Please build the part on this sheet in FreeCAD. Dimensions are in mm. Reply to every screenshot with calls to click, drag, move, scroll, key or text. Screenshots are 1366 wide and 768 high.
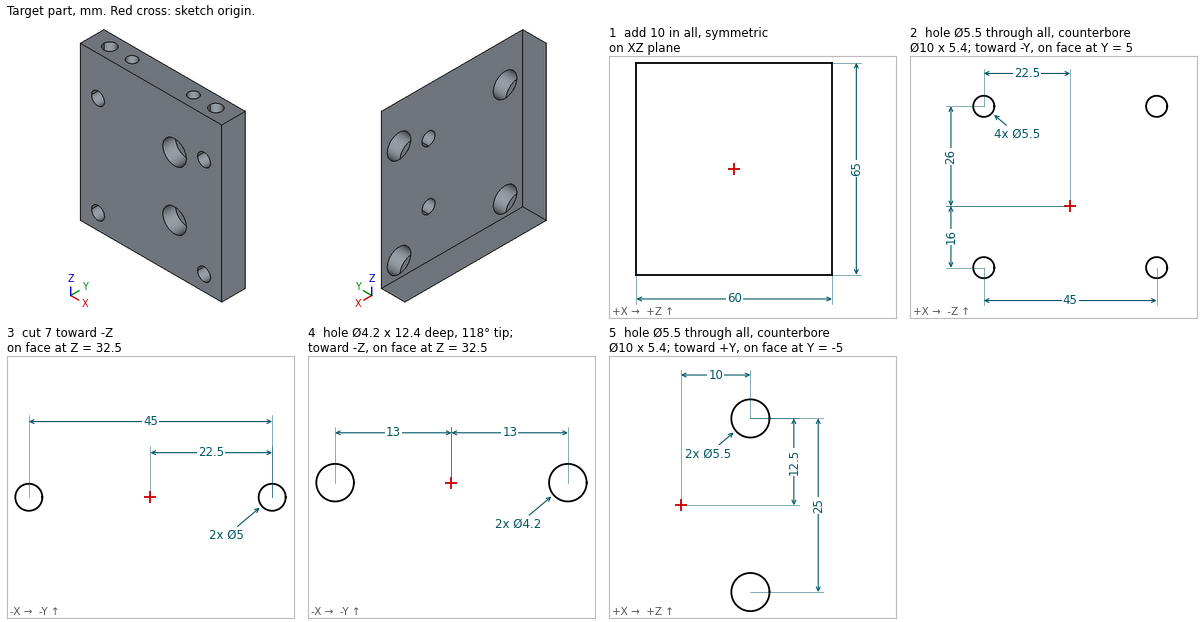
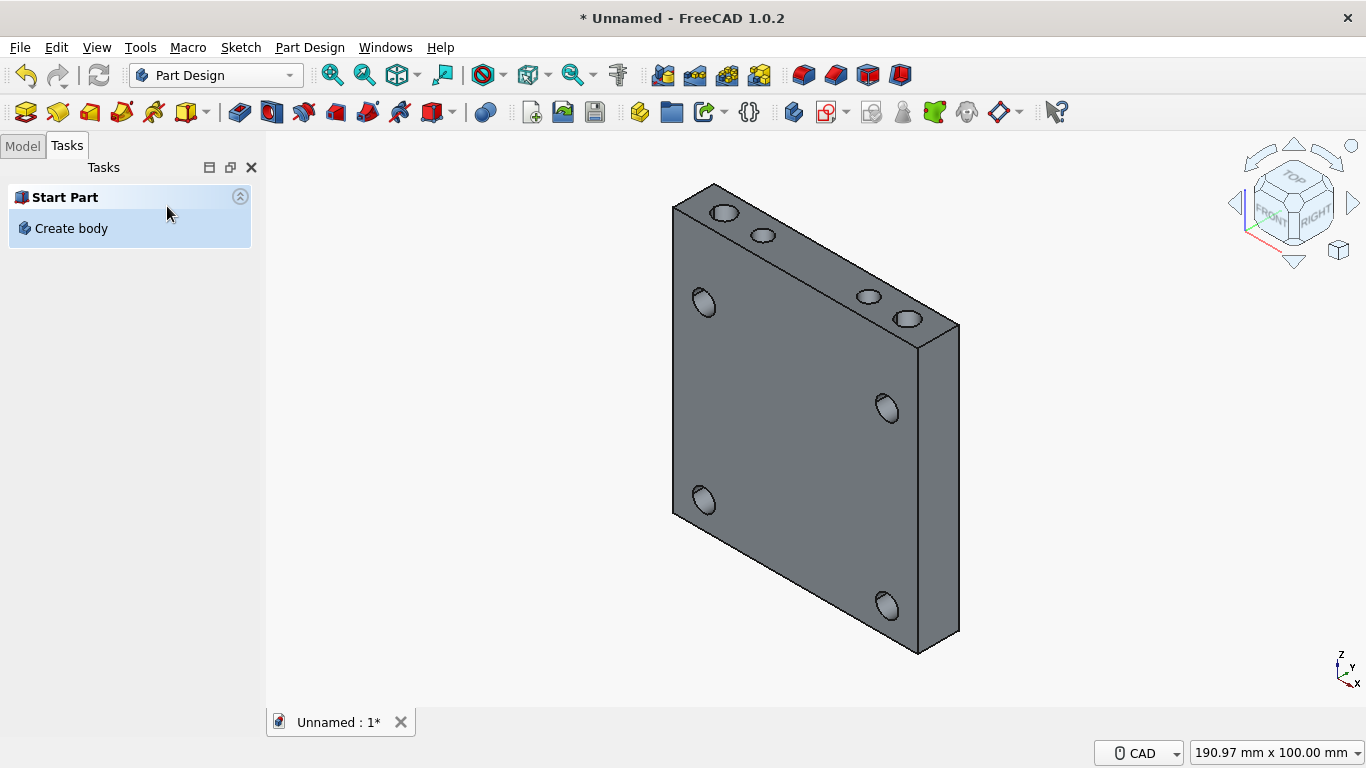
click(796, 430)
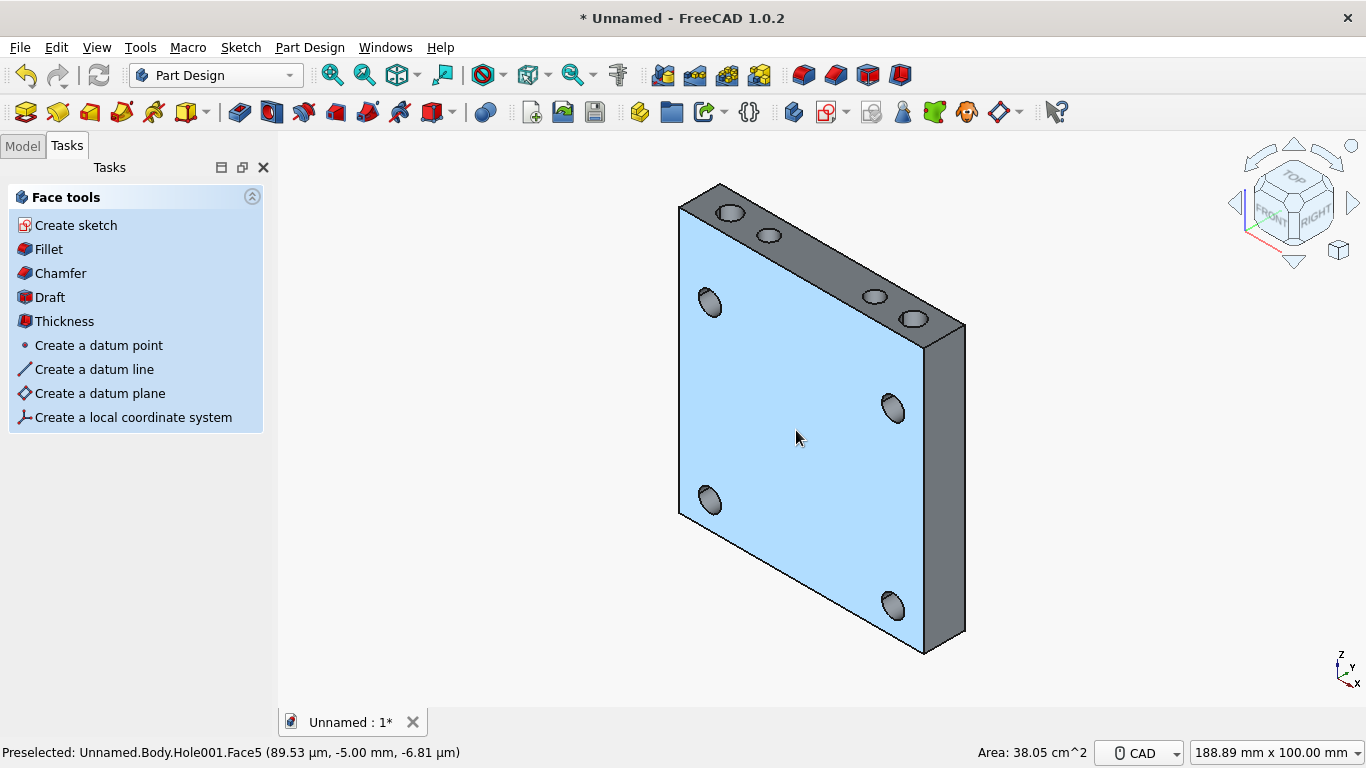
click(826, 112)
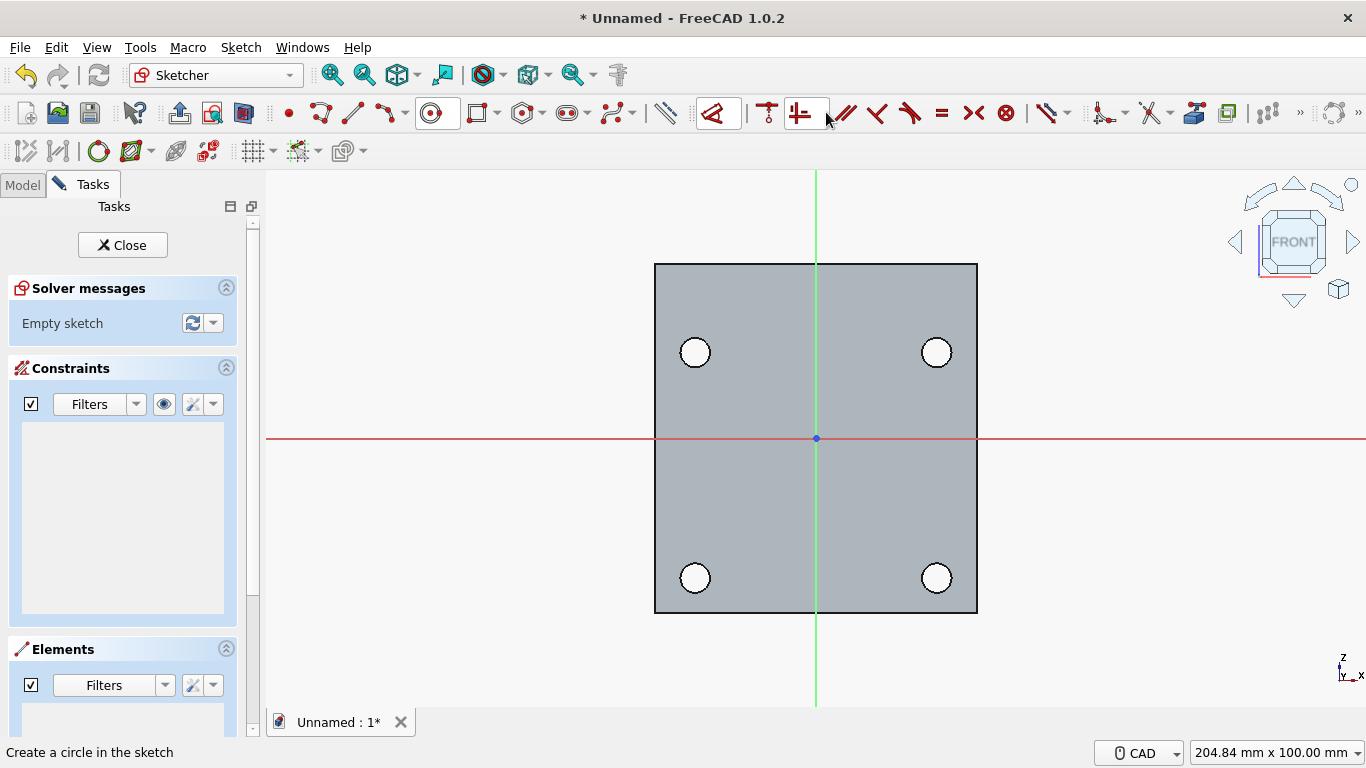
scroll(934, 439, up, 4)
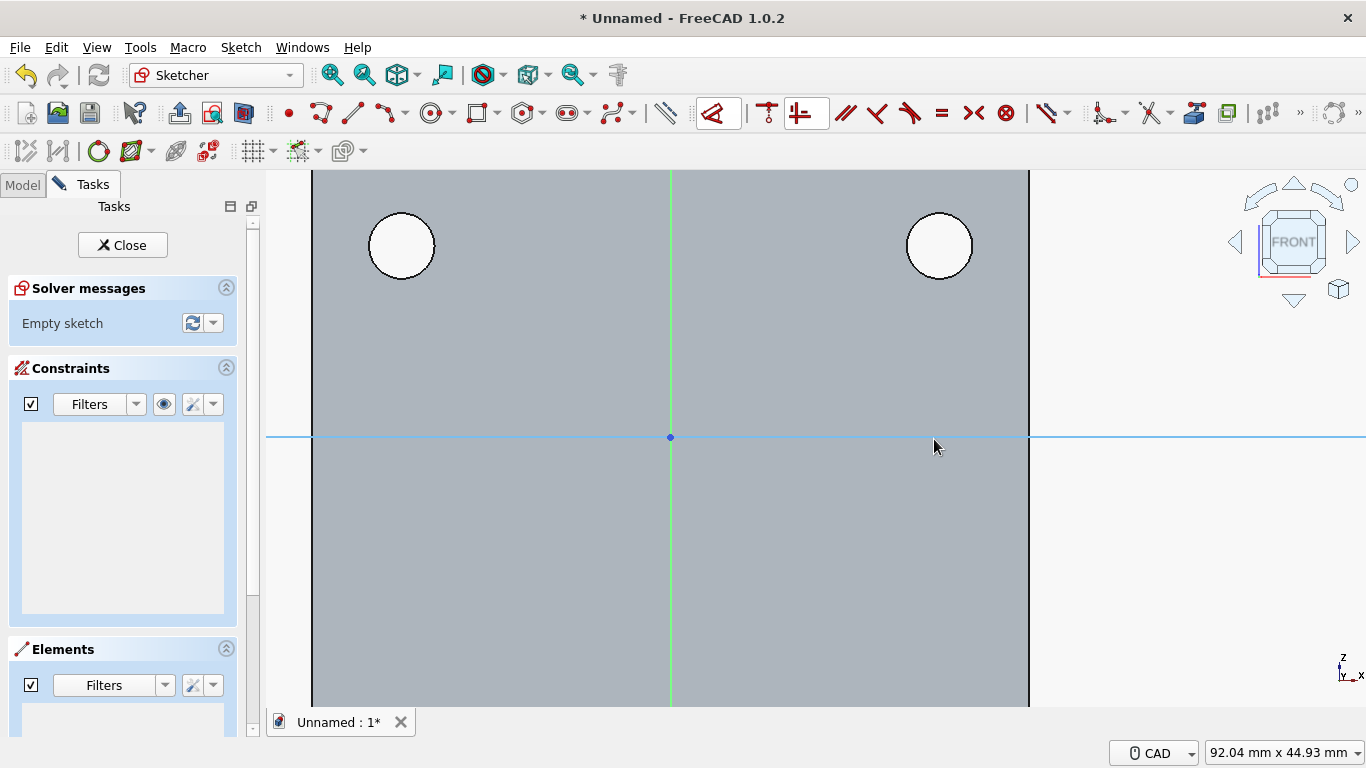
key(g)
key(c)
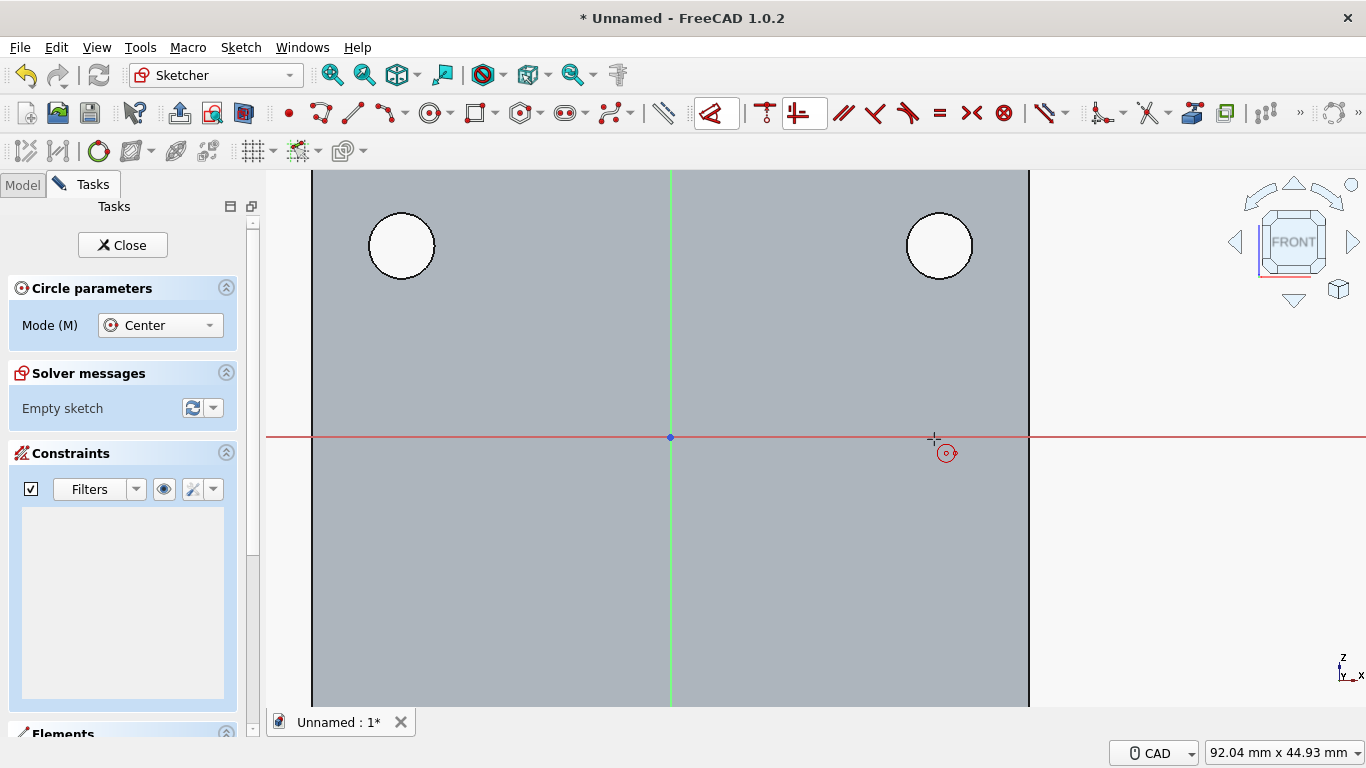
click(790, 288)
click(813, 265)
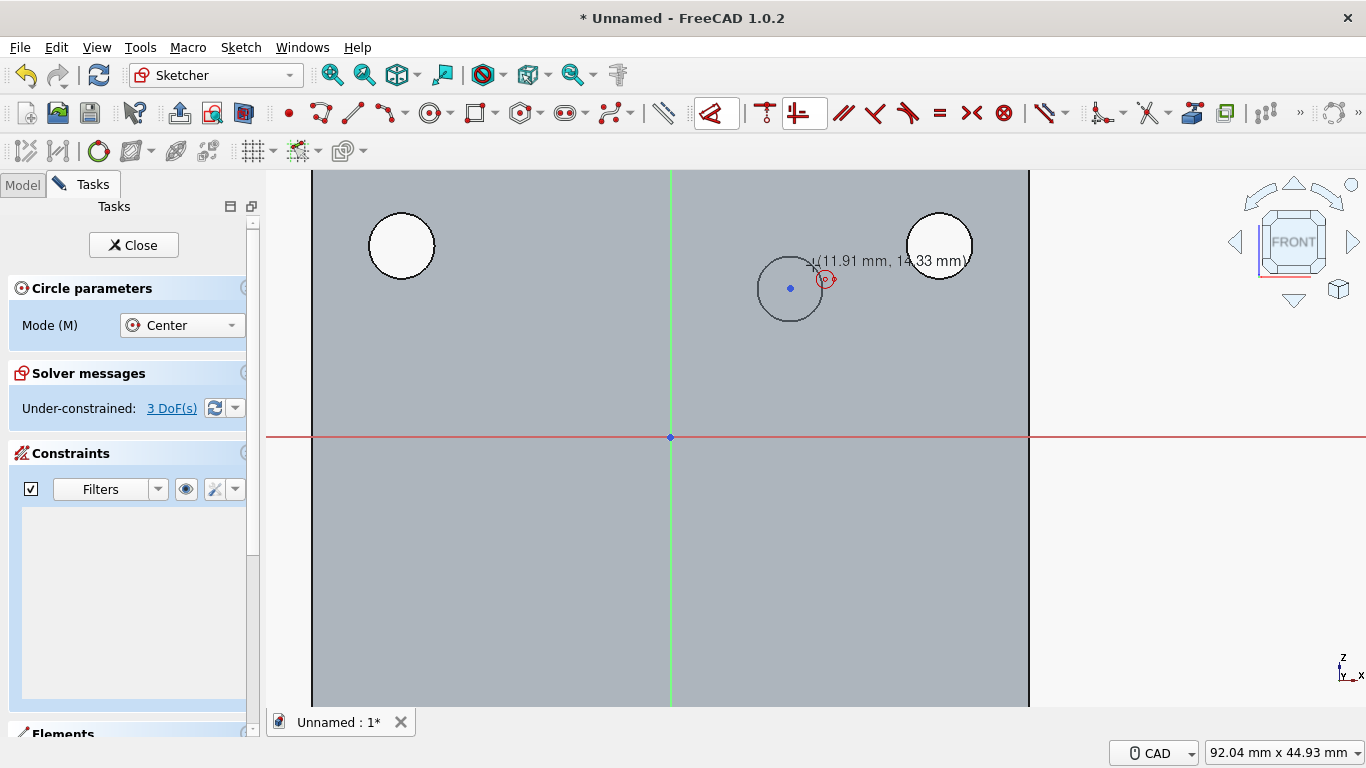
click(790, 587)
click(813, 563)
key(Escape)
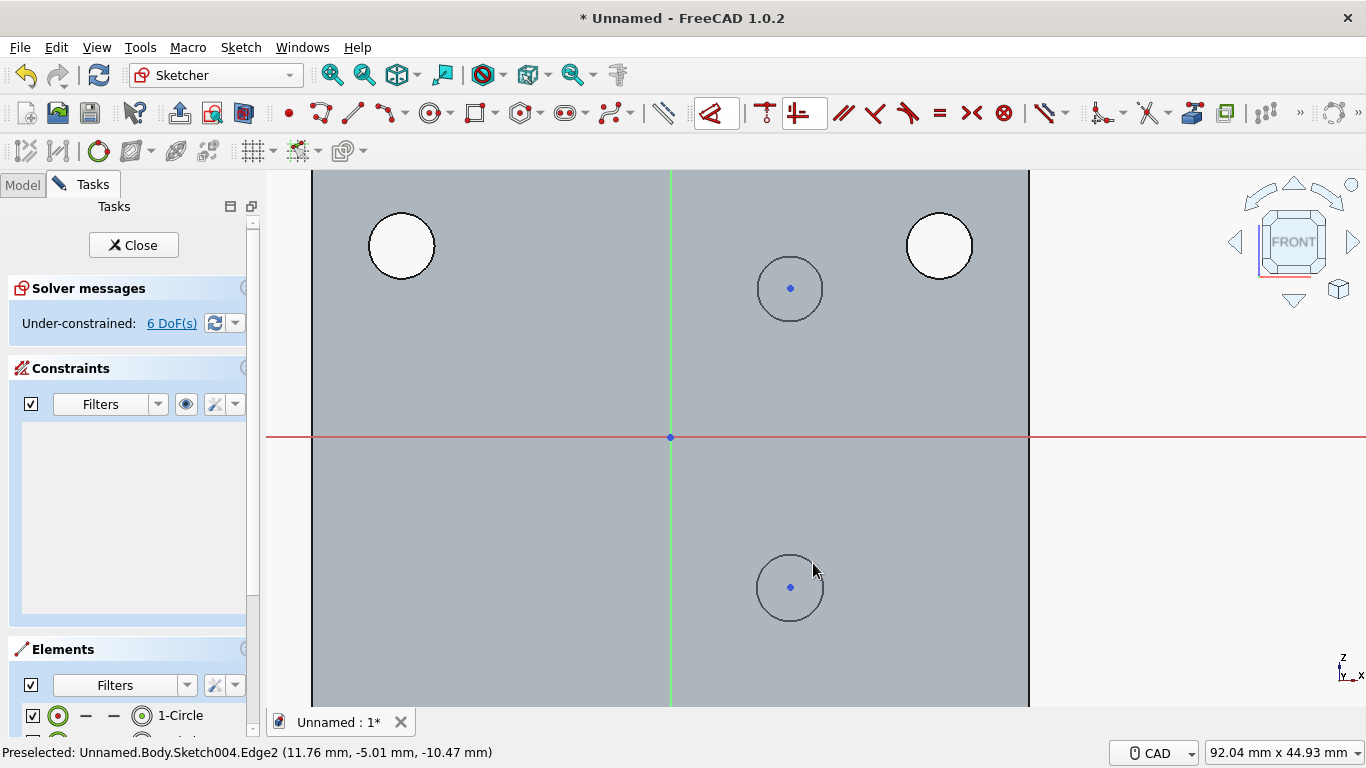
click(813, 266)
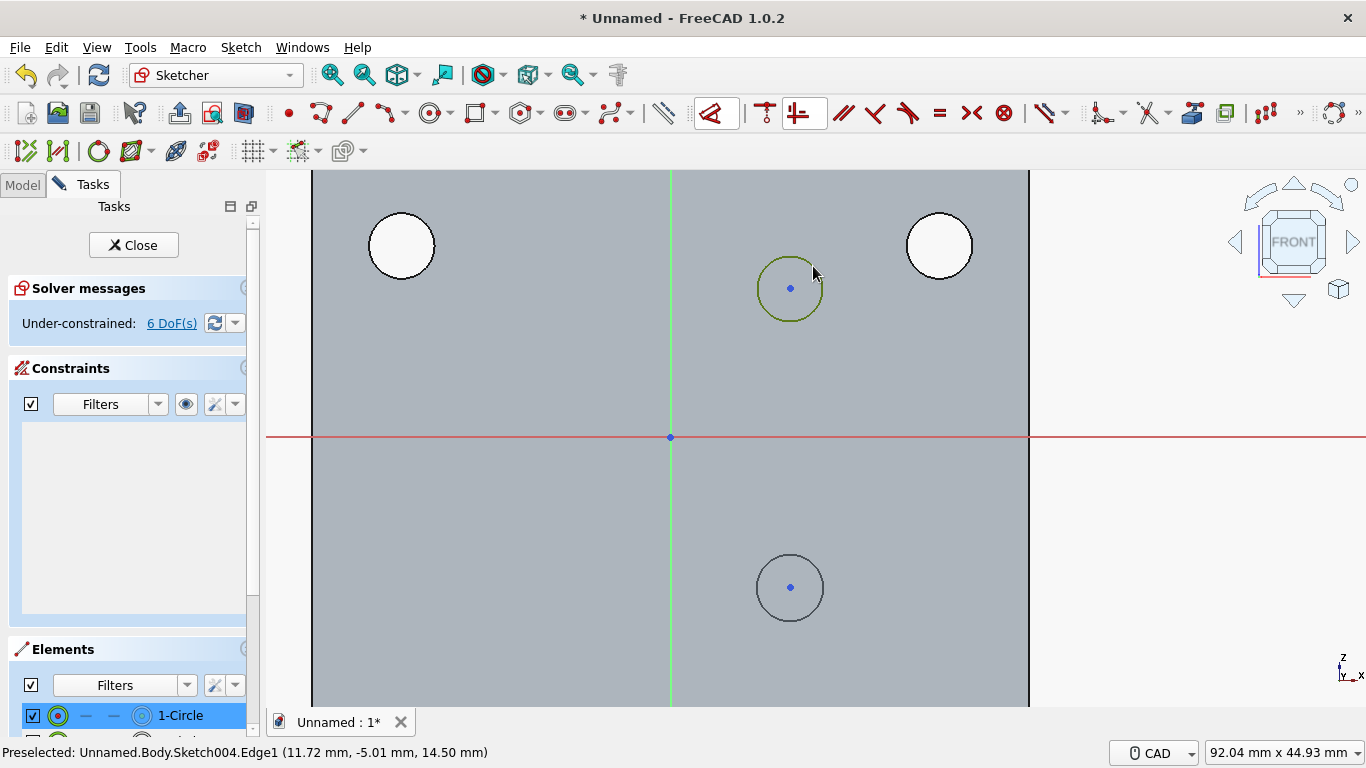
click(813, 564)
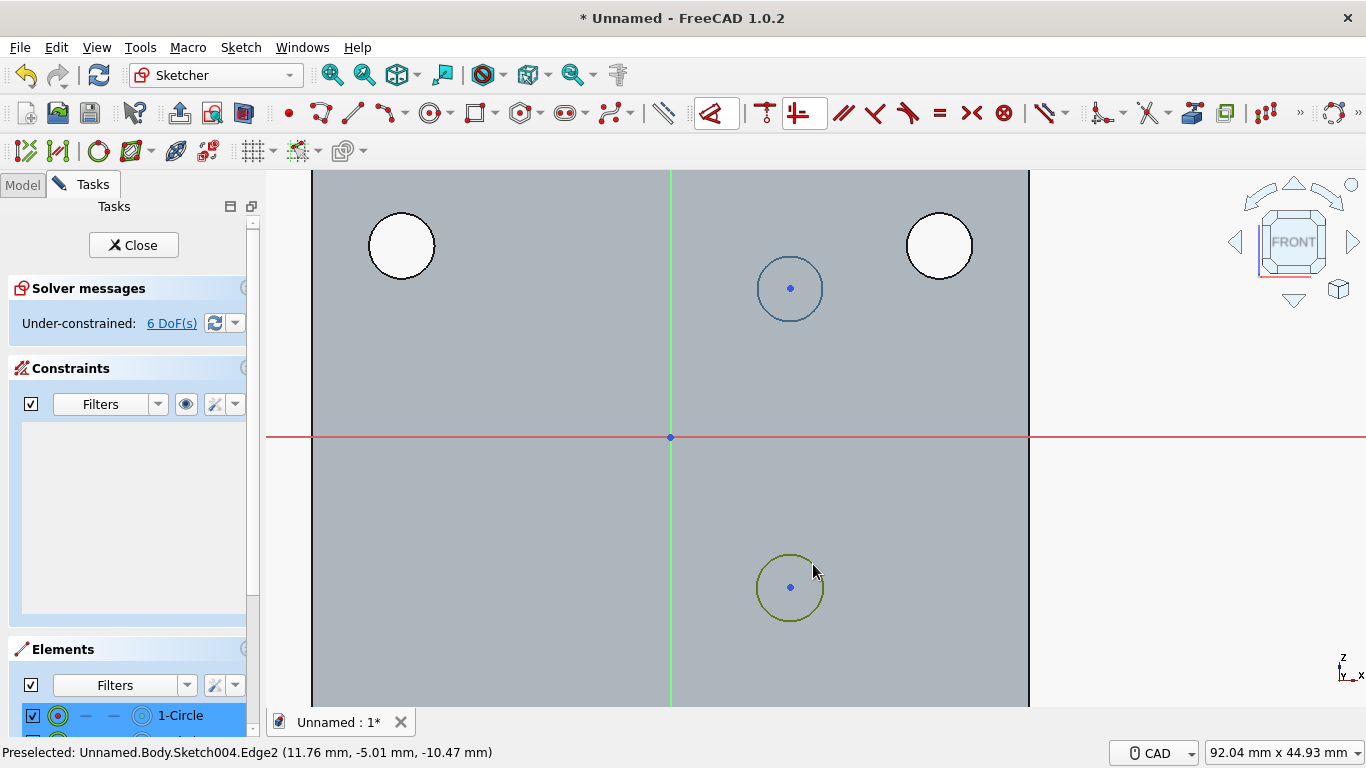
key(e)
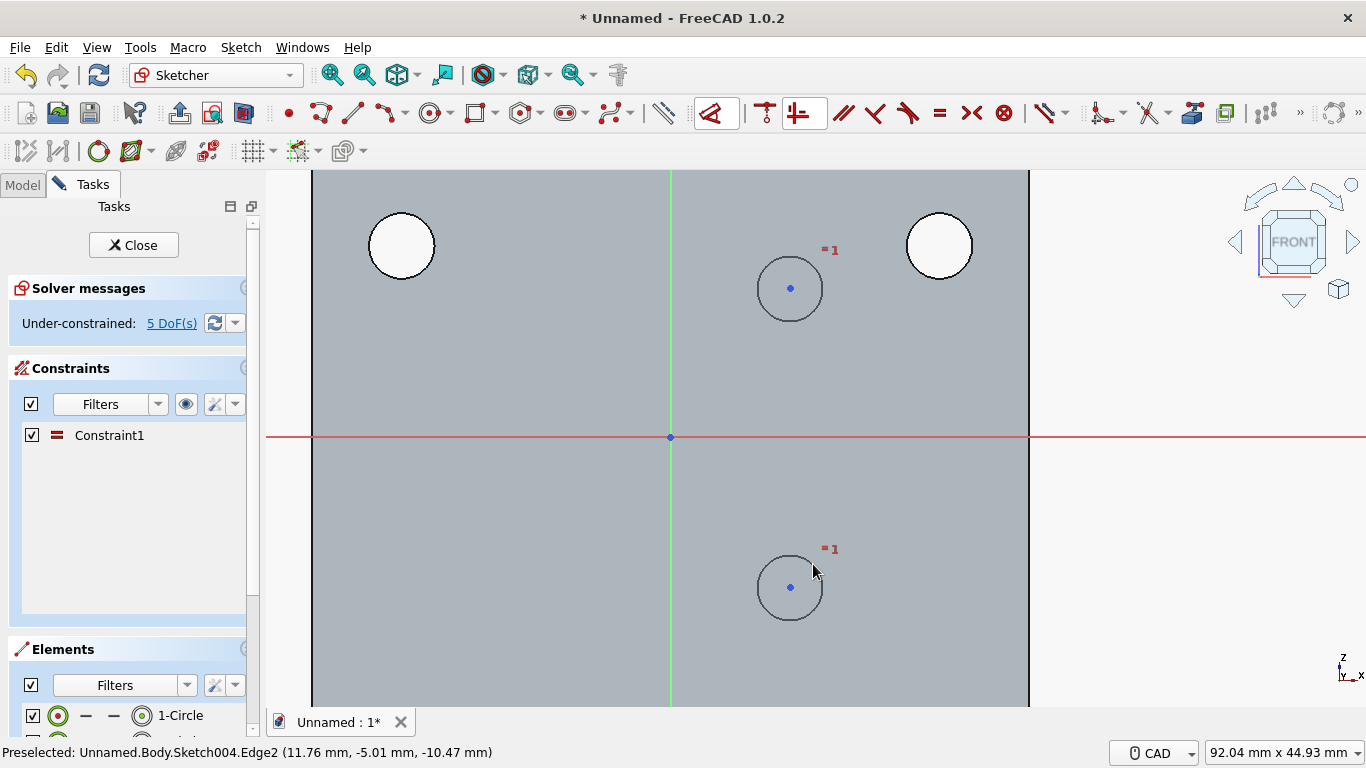
click(790, 289)